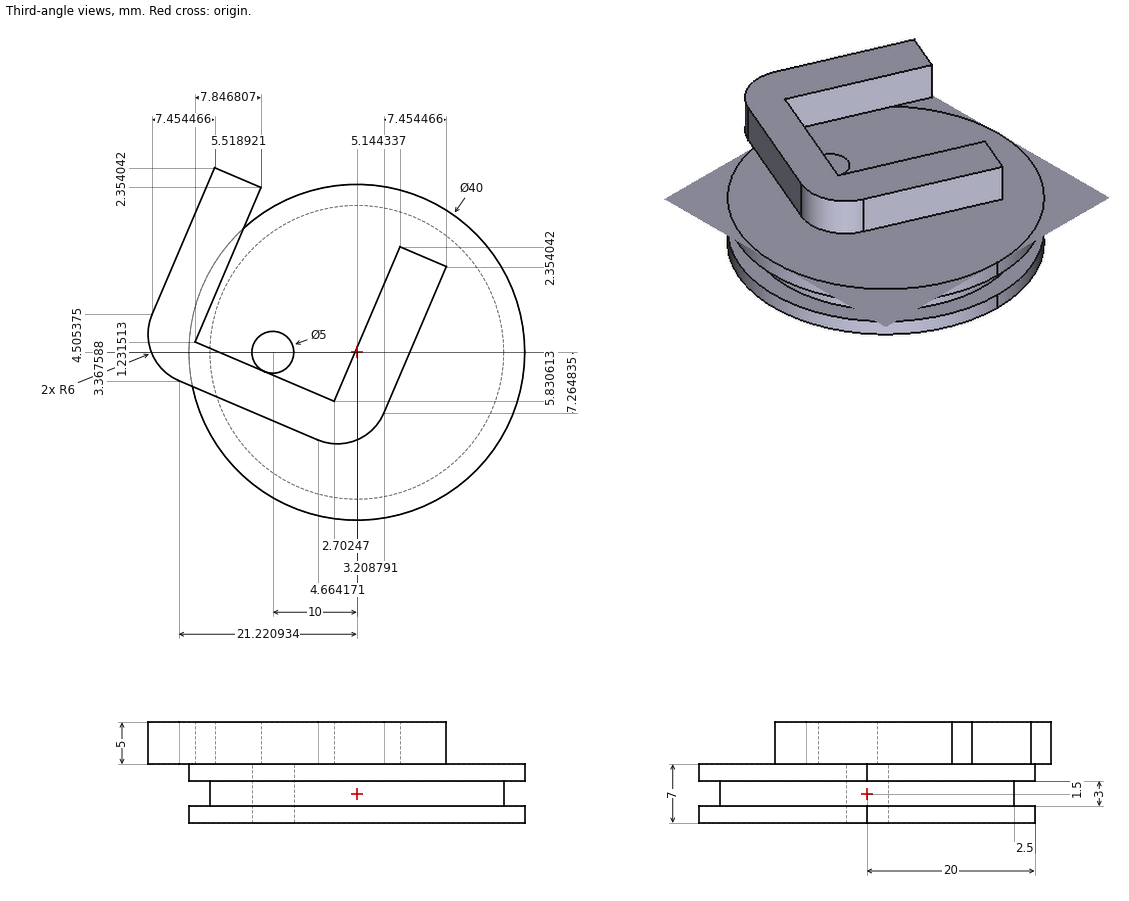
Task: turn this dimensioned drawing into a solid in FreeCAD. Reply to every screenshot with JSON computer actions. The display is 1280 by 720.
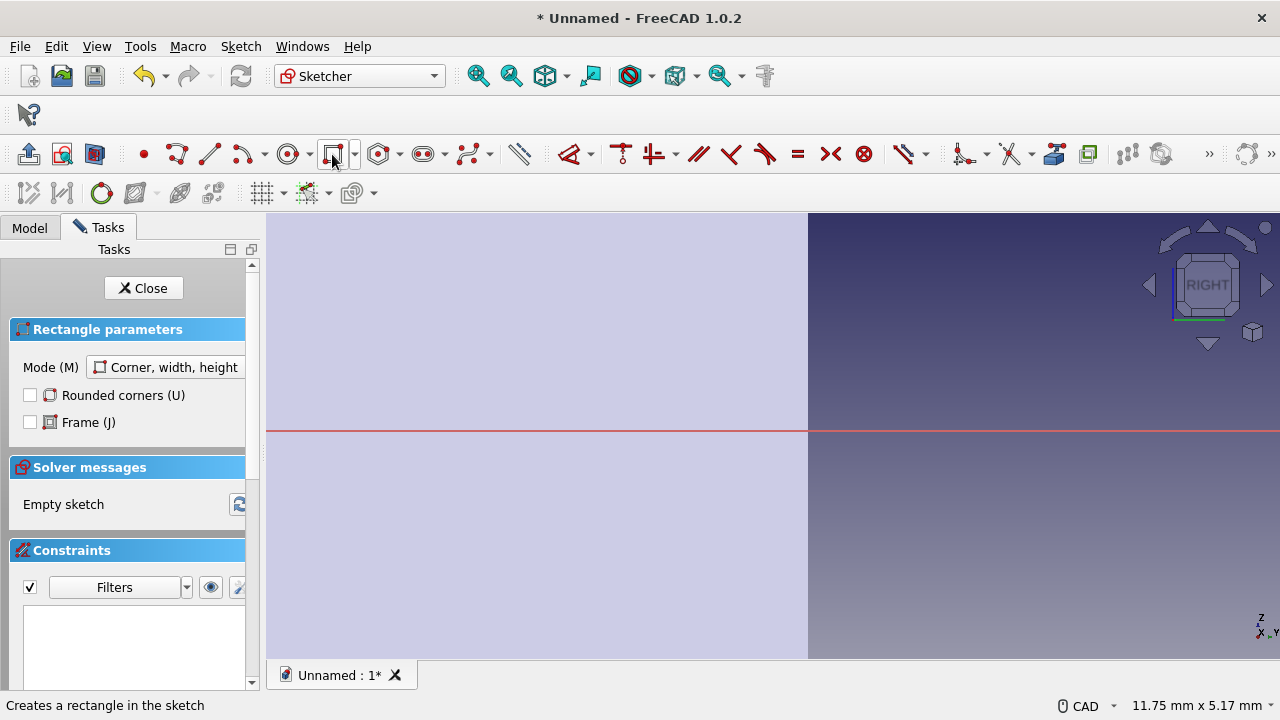
{"action": "left_click", "coordinate": [593, 302]}
{"action": "left_click", "coordinate": [808, 560]}
{"action": "key", "text": "Escape"}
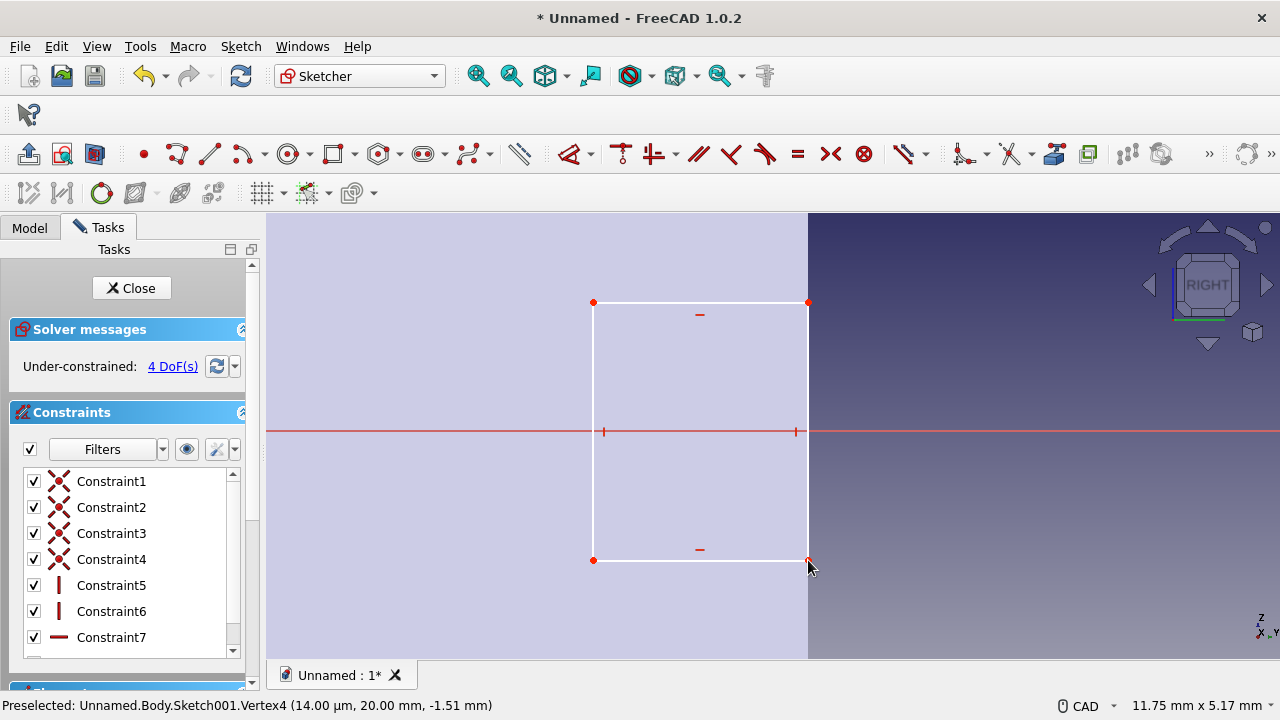
{"action": "left_click", "coordinate": [568, 154]}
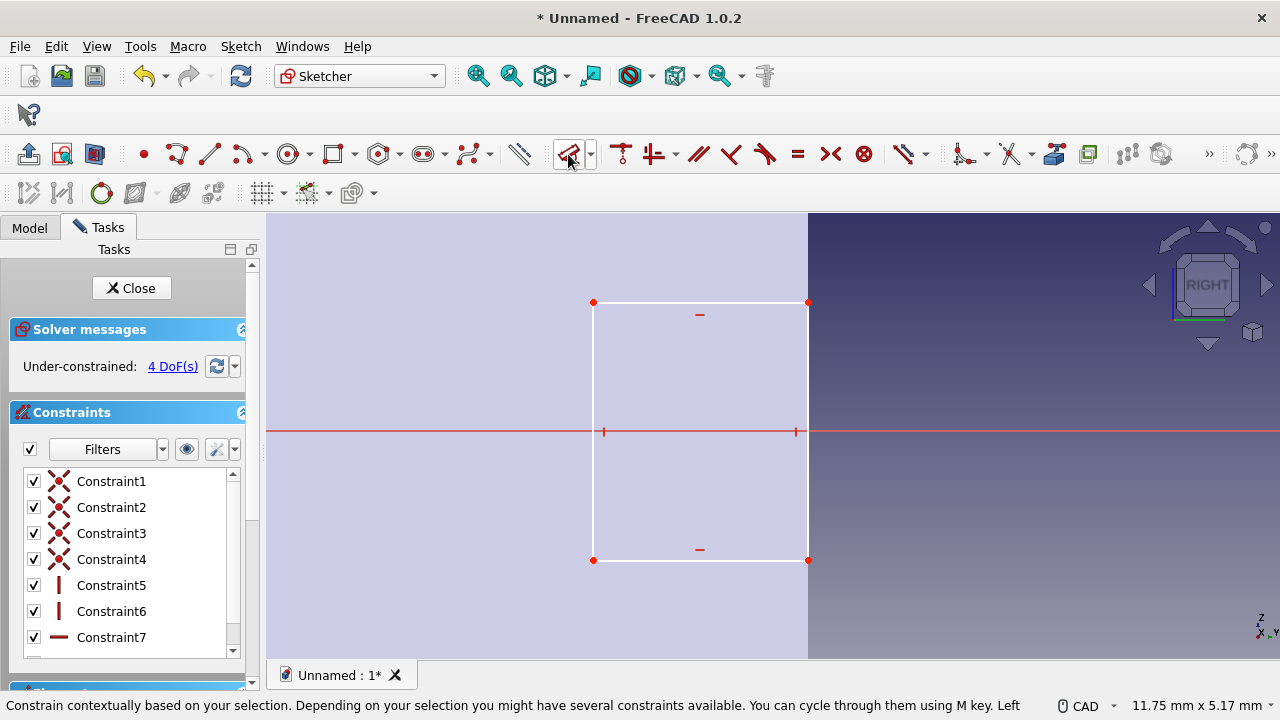
{"action": "left_click", "coordinate": [593, 380]}
{"action": "left_click", "coordinate": [559, 373]}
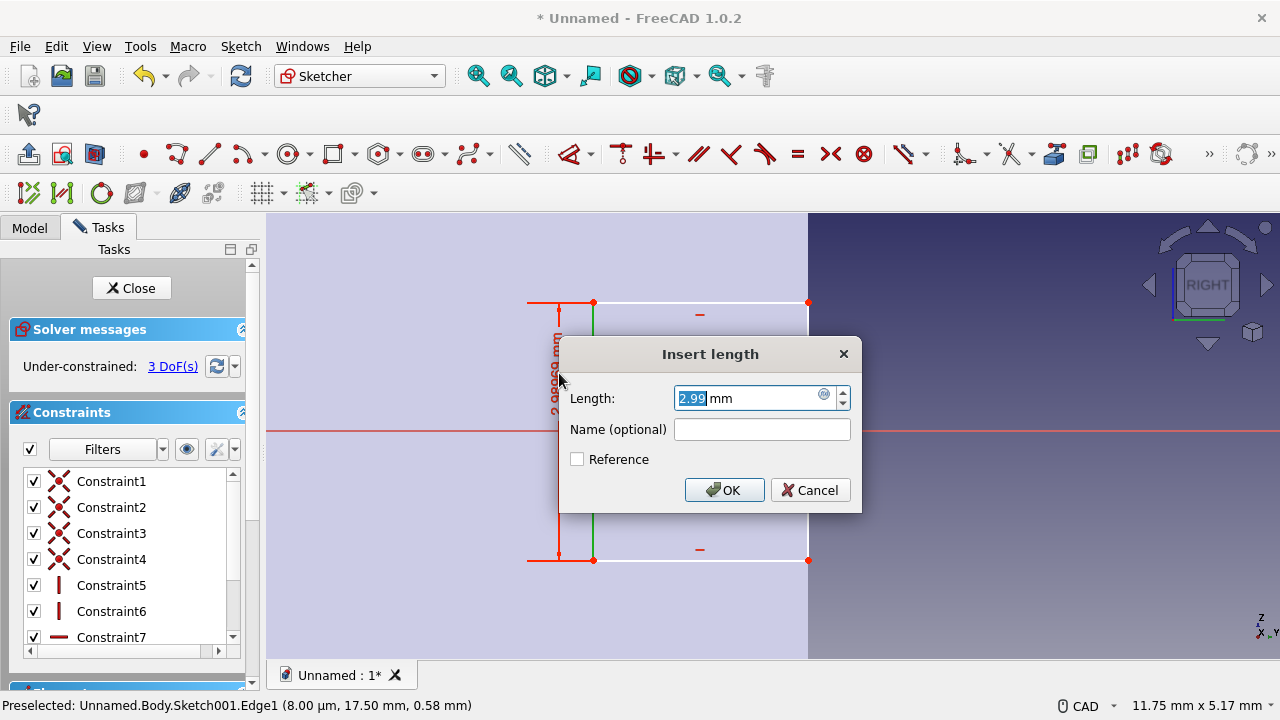
{"action": "type", "text": "3"}
{"action": "key", "text": "Return"}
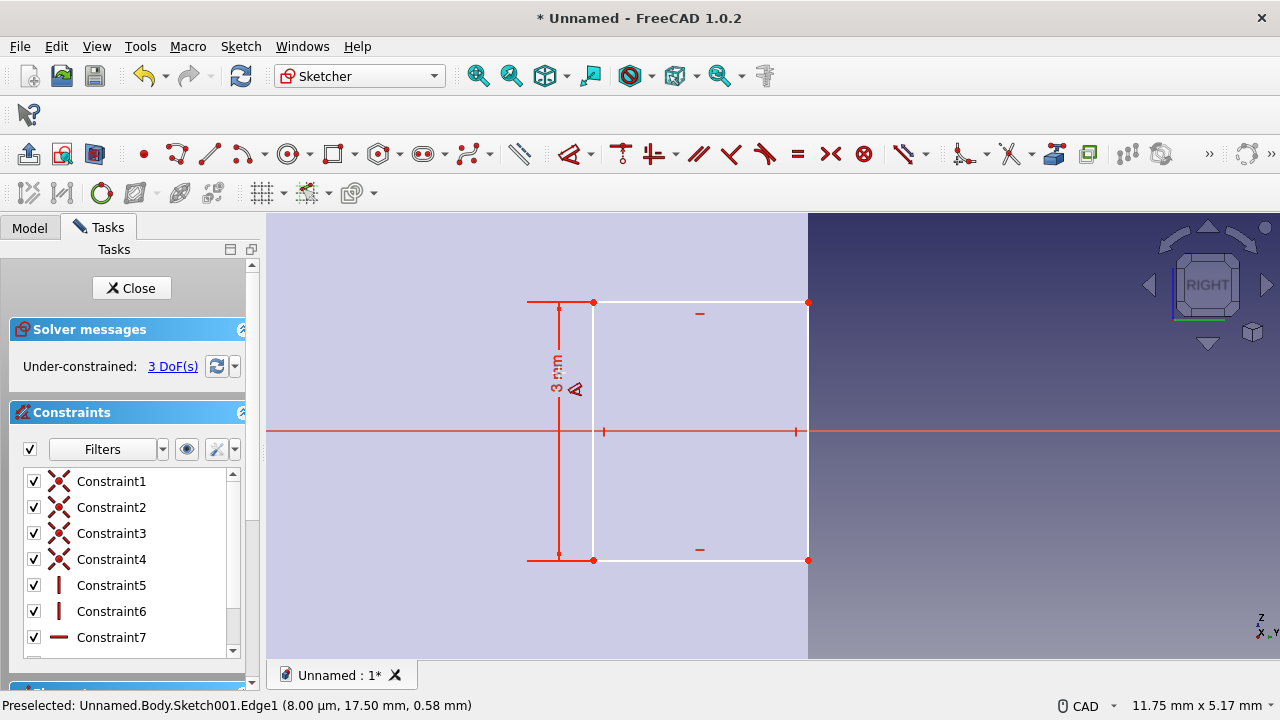
{"action": "left_click", "coordinate": [658, 561]}
{"action": "left_click", "coordinate": [701, 595]}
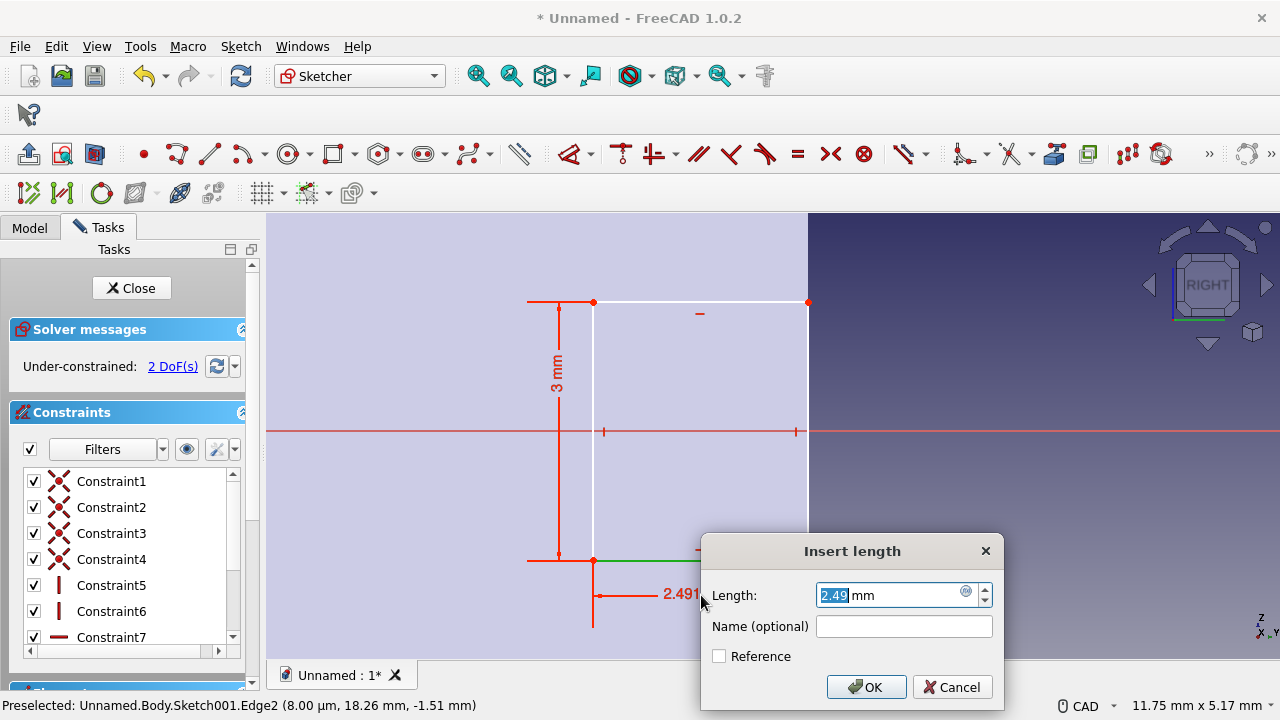
{"action": "type", "text": "2.5"}
{"action": "key", "text": "Return"}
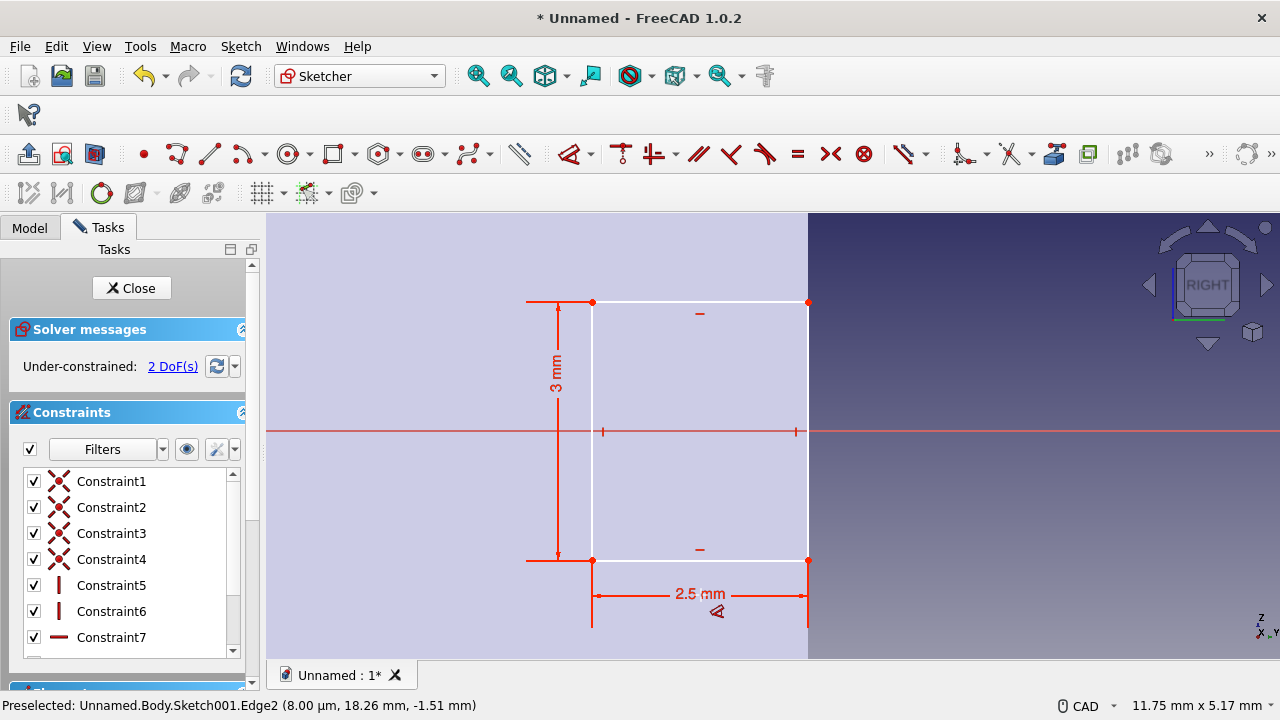
{"action": "left_click", "coordinate": [808, 561]}
{"action": "left_click", "coordinate": [551, 595]}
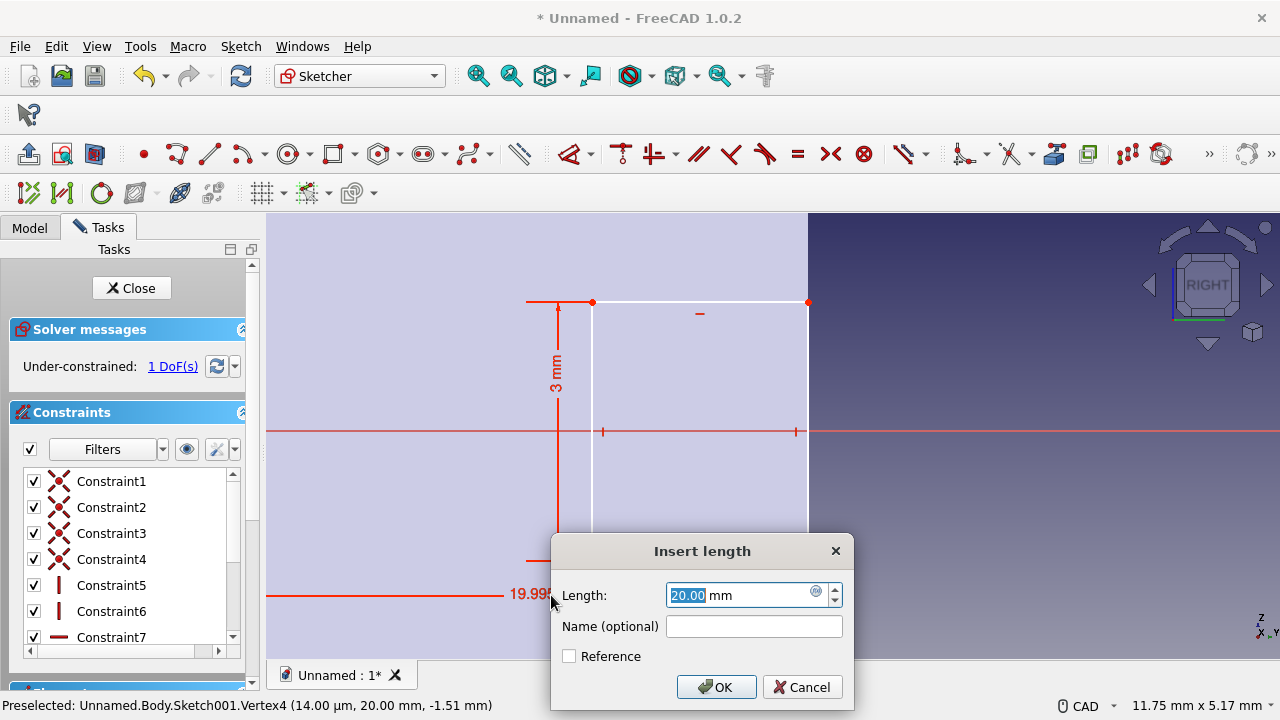
{"action": "type", "text": "20"}
{"action": "key", "text": "Return"}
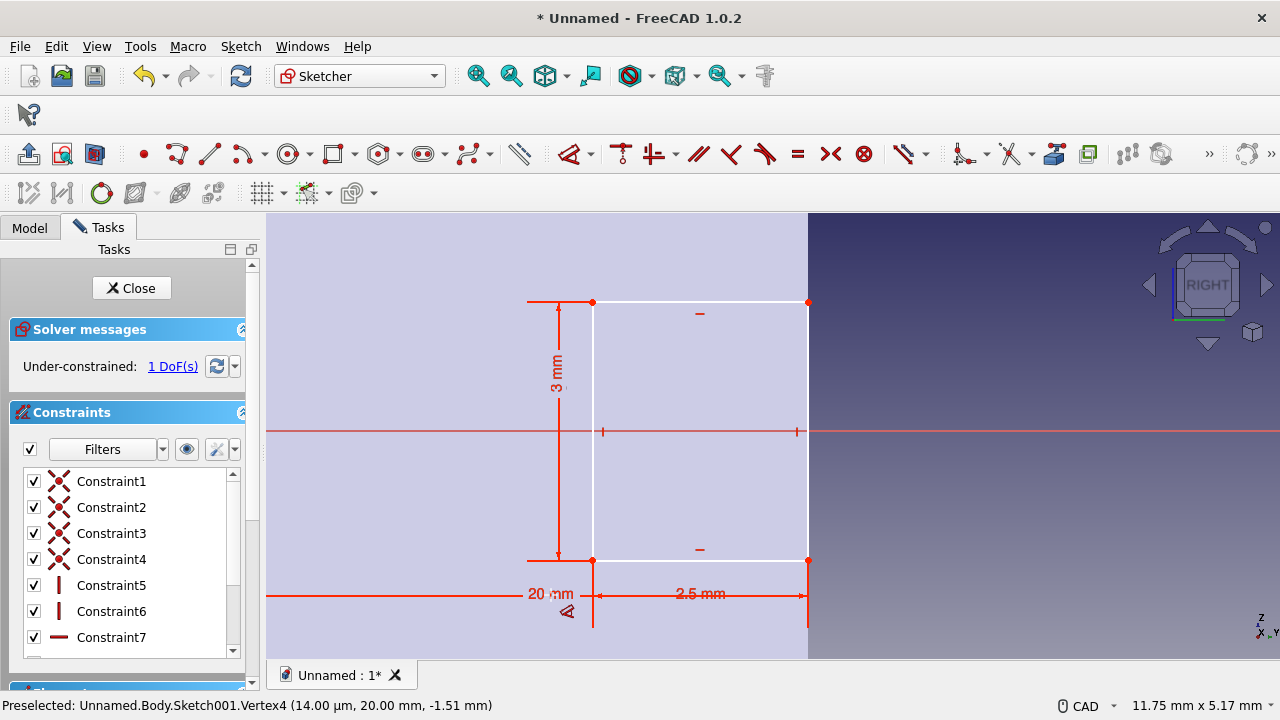
{"action": "left_click", "coordinate": [593, 302]}
{"action": "left_click", "coordinate": [627, 337]}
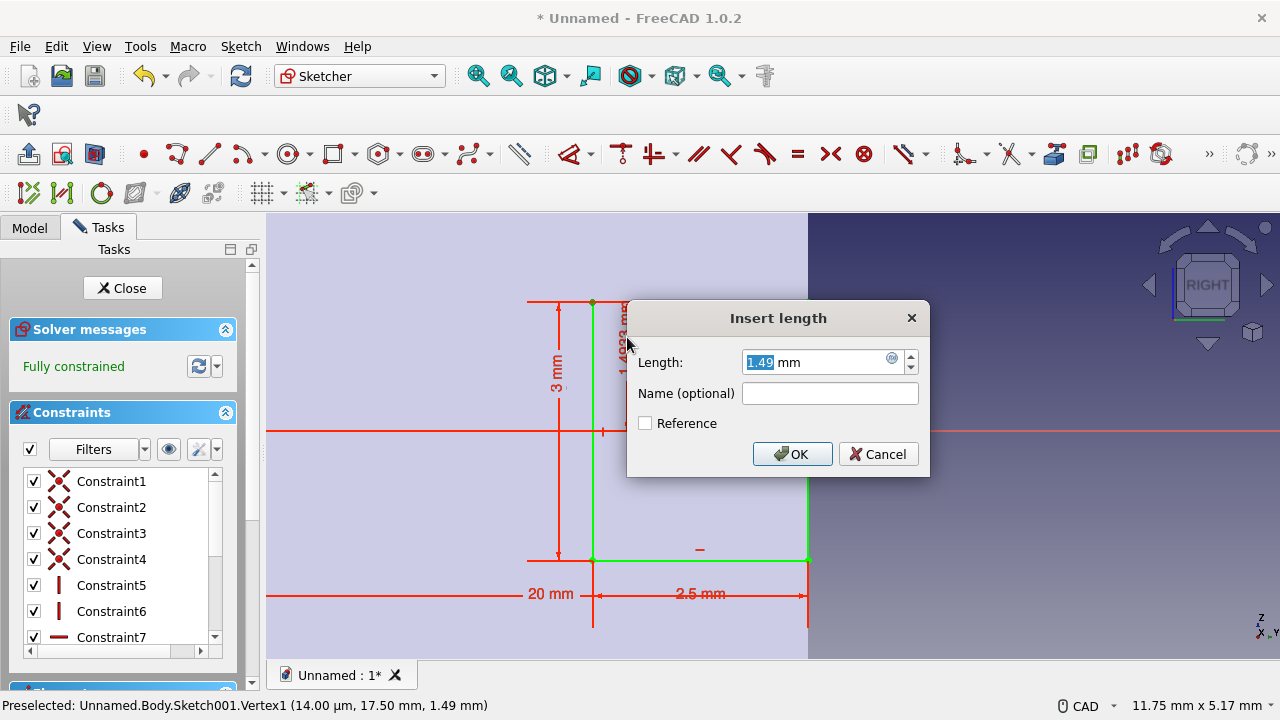
{"action": "type", "text": "1.5"}
{"action": "key", "text": "Return"}
{"action": "key", "text": "Escape"}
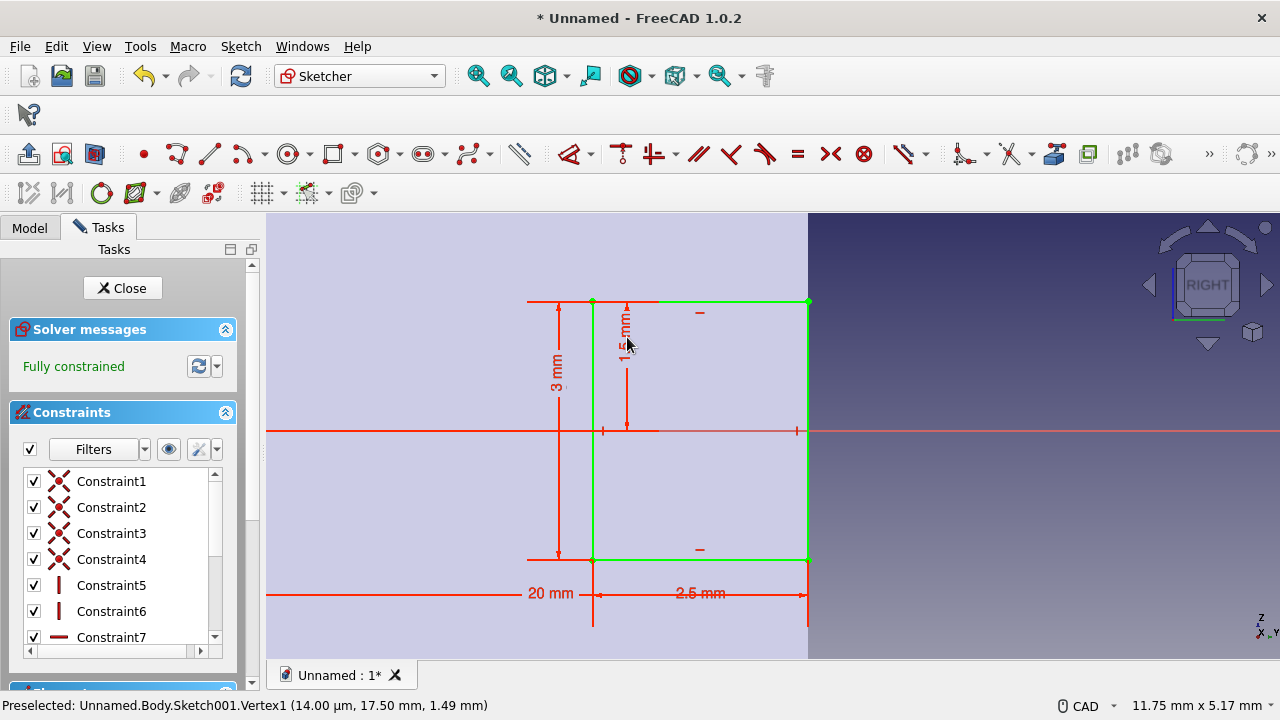
{"action": "left_click", "coordinate": [123, 288]}